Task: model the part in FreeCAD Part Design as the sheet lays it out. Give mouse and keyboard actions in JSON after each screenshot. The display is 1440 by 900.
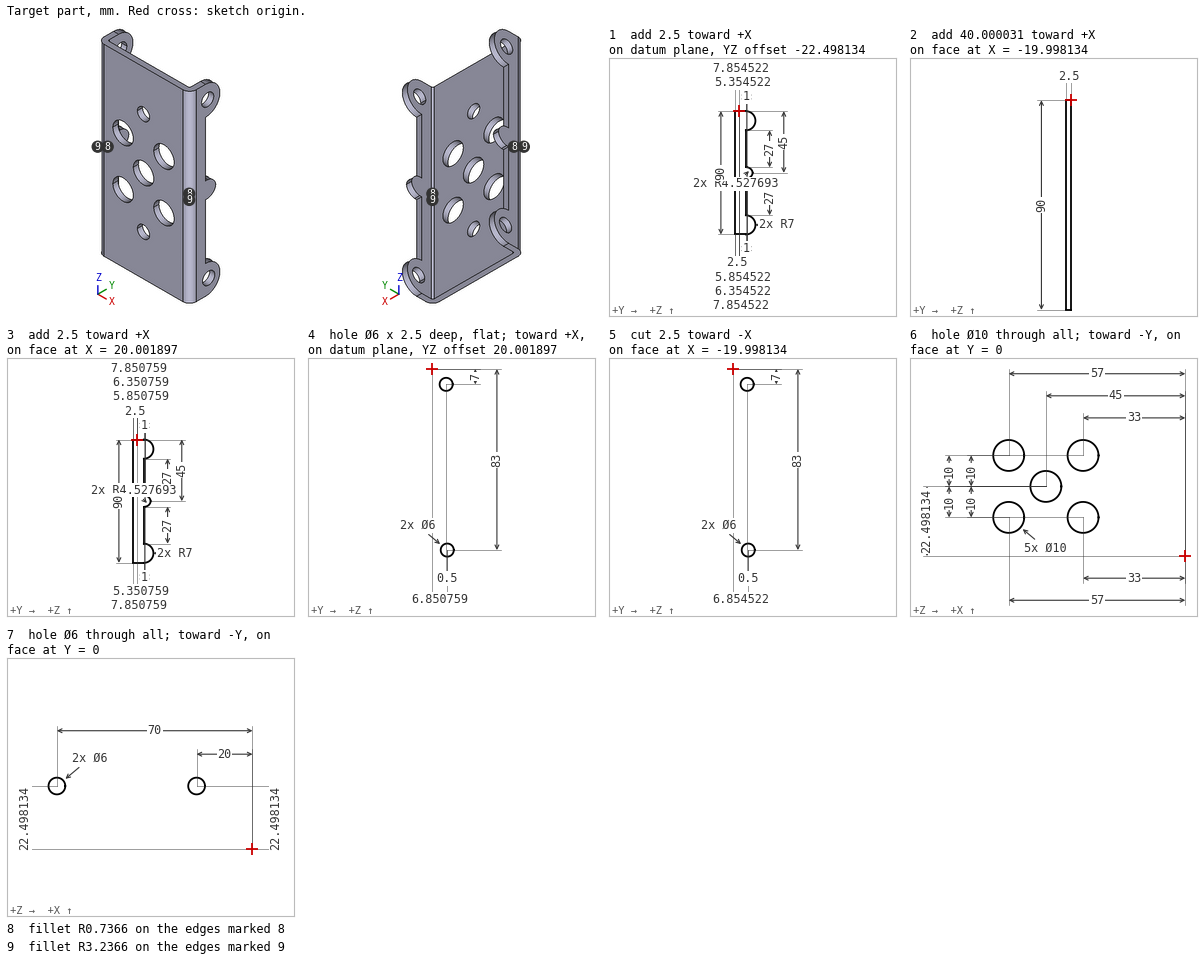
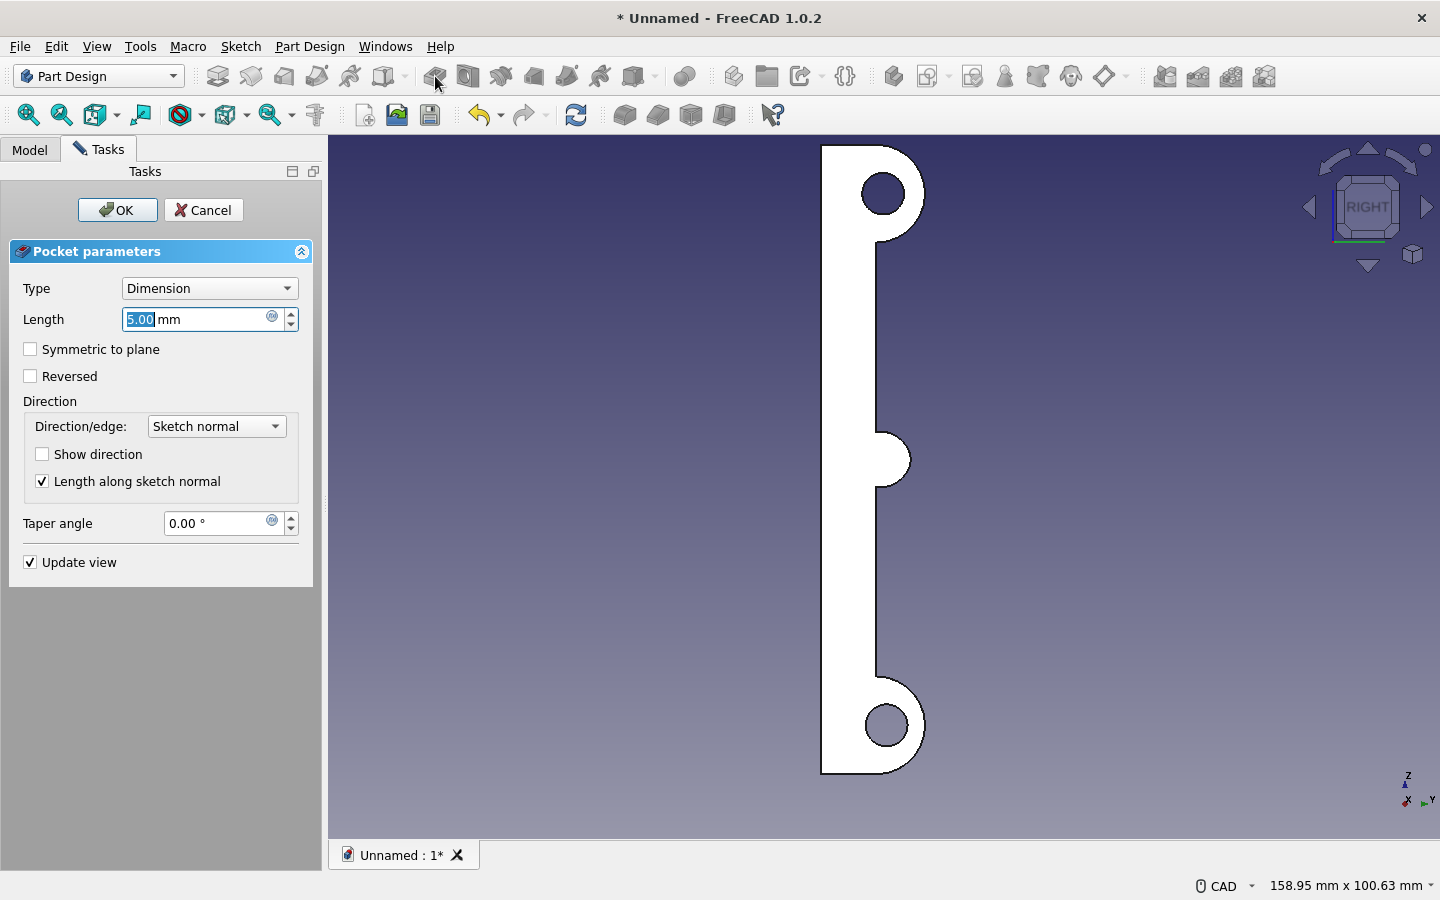
{"action": "type", "text": "2.5"}
{"action": "key", "text": "Tab"}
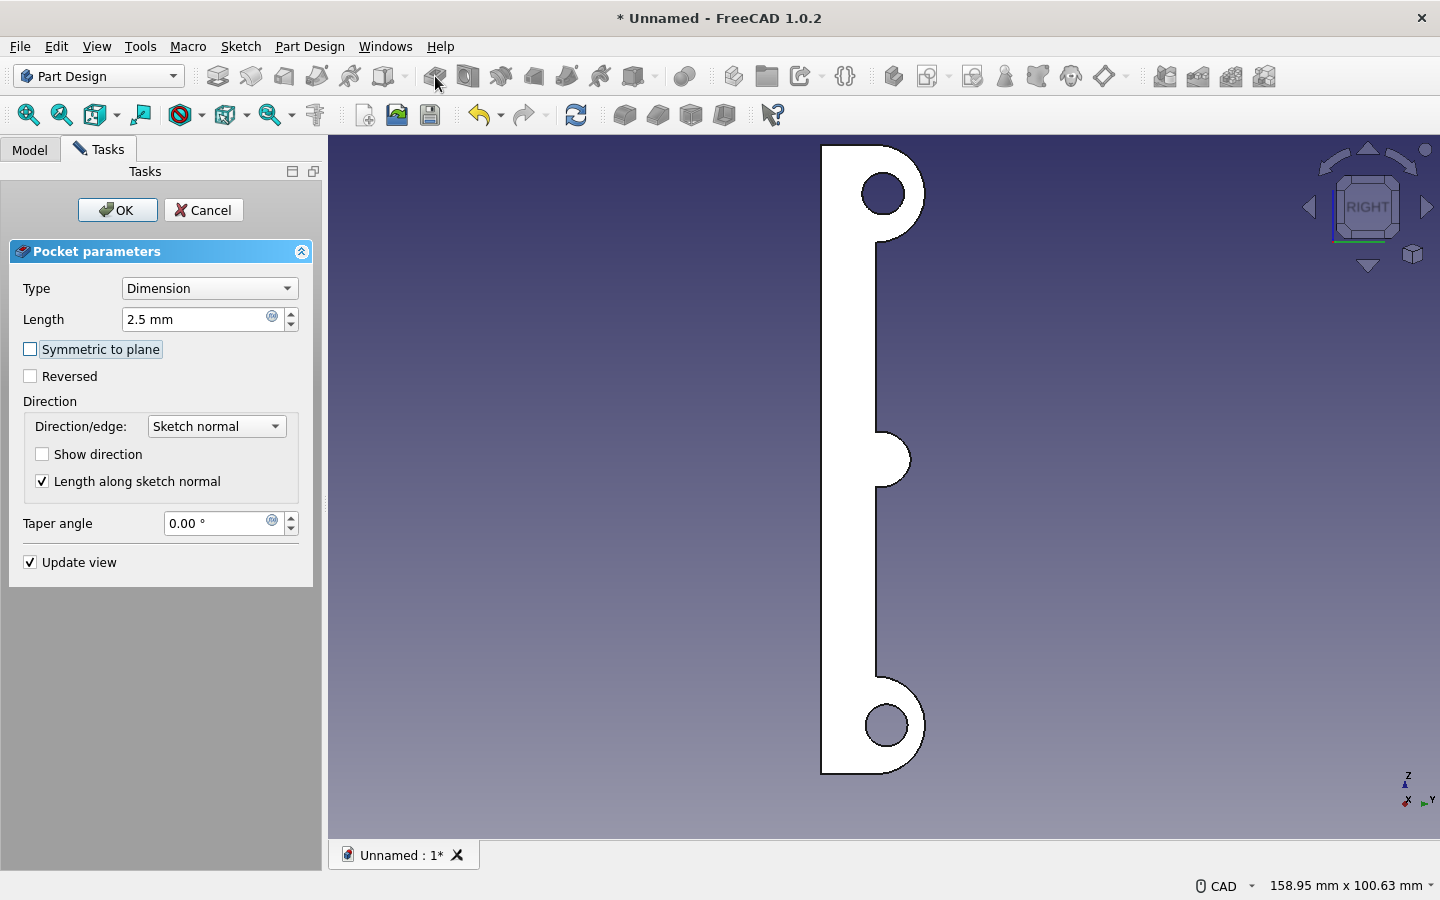
{"action": "left_click", "coordinate": [118, 210]}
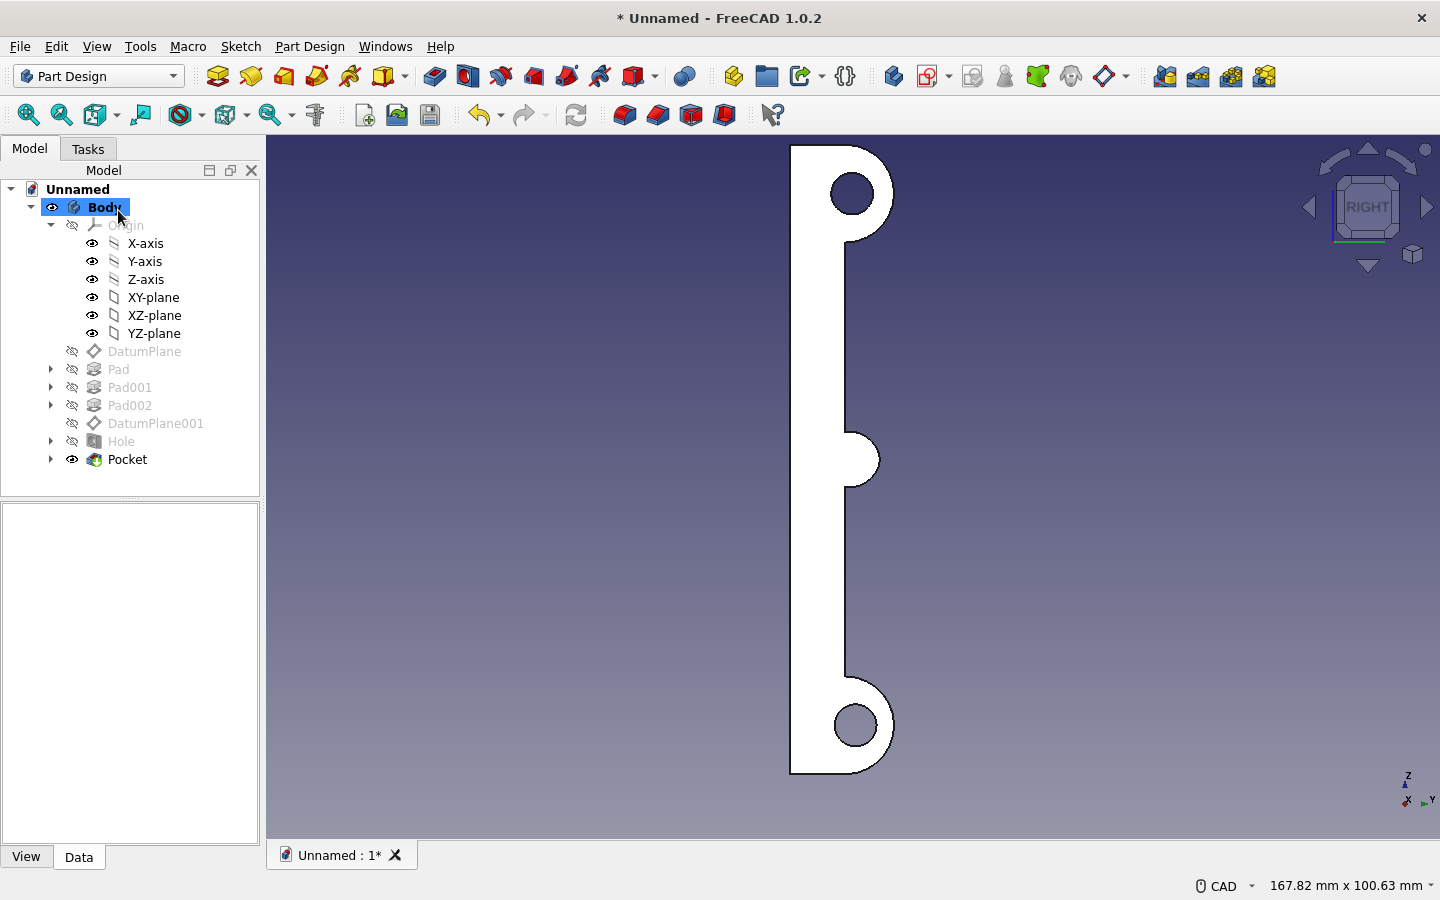
{"action": "key", "text": "4"}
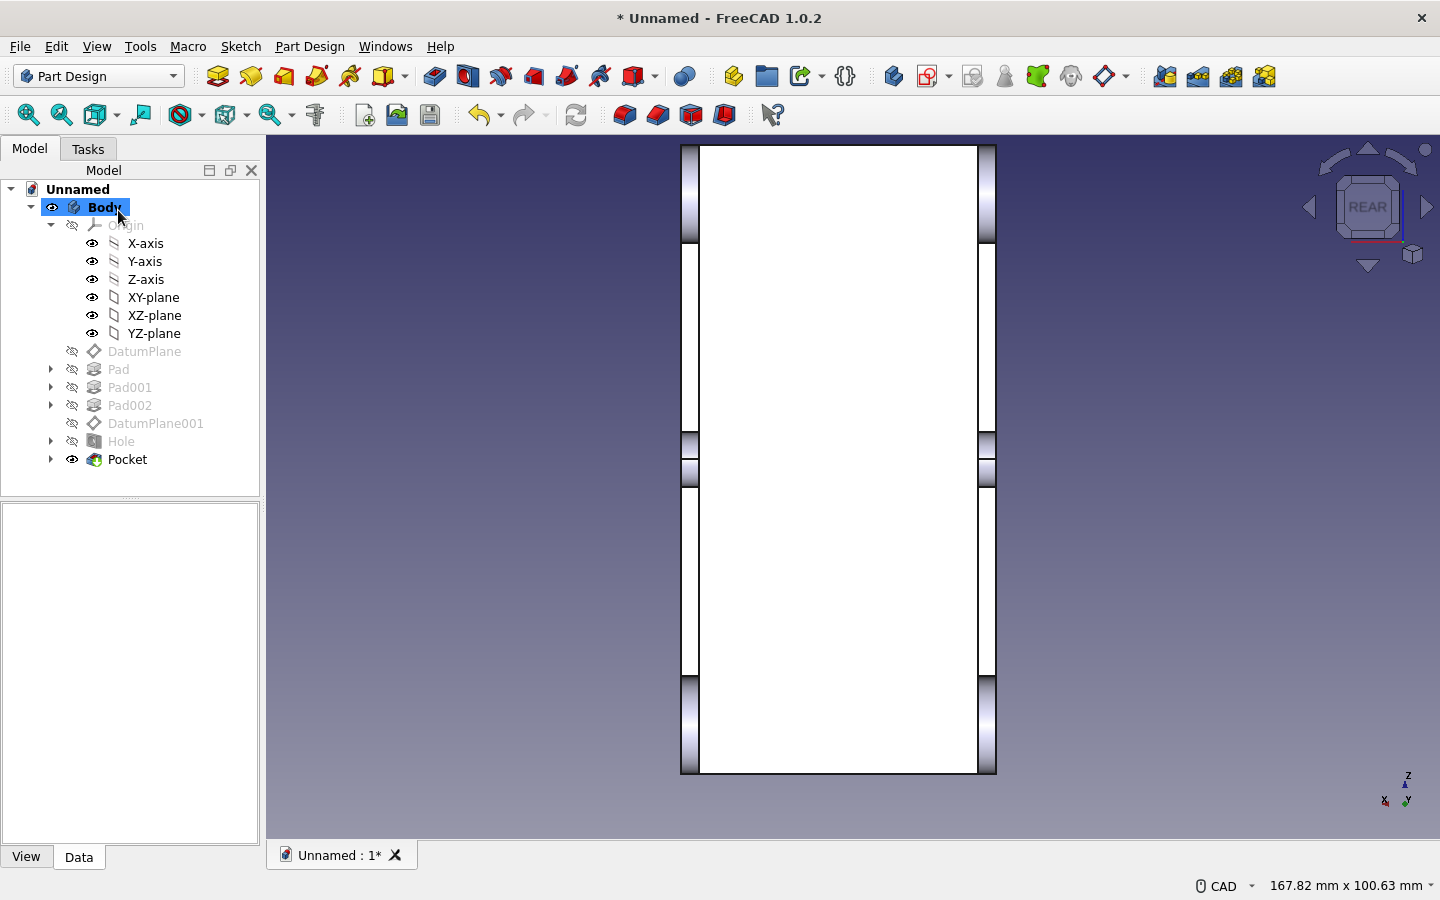
{"action": "left_click", "coordinate": [838, 369]}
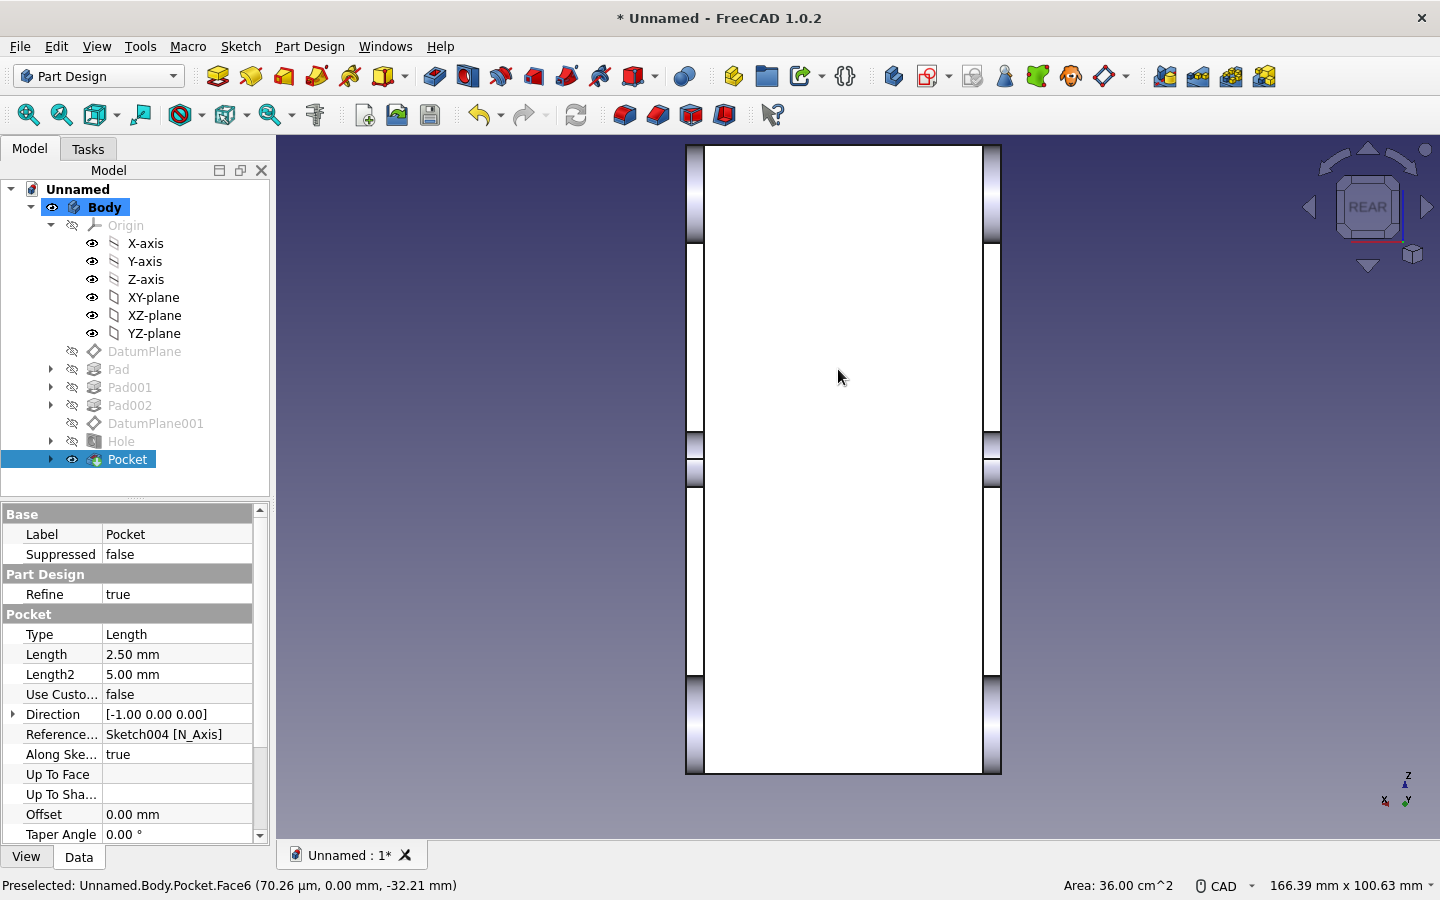
{"action": "left_click", "coordinate": [926, 76]}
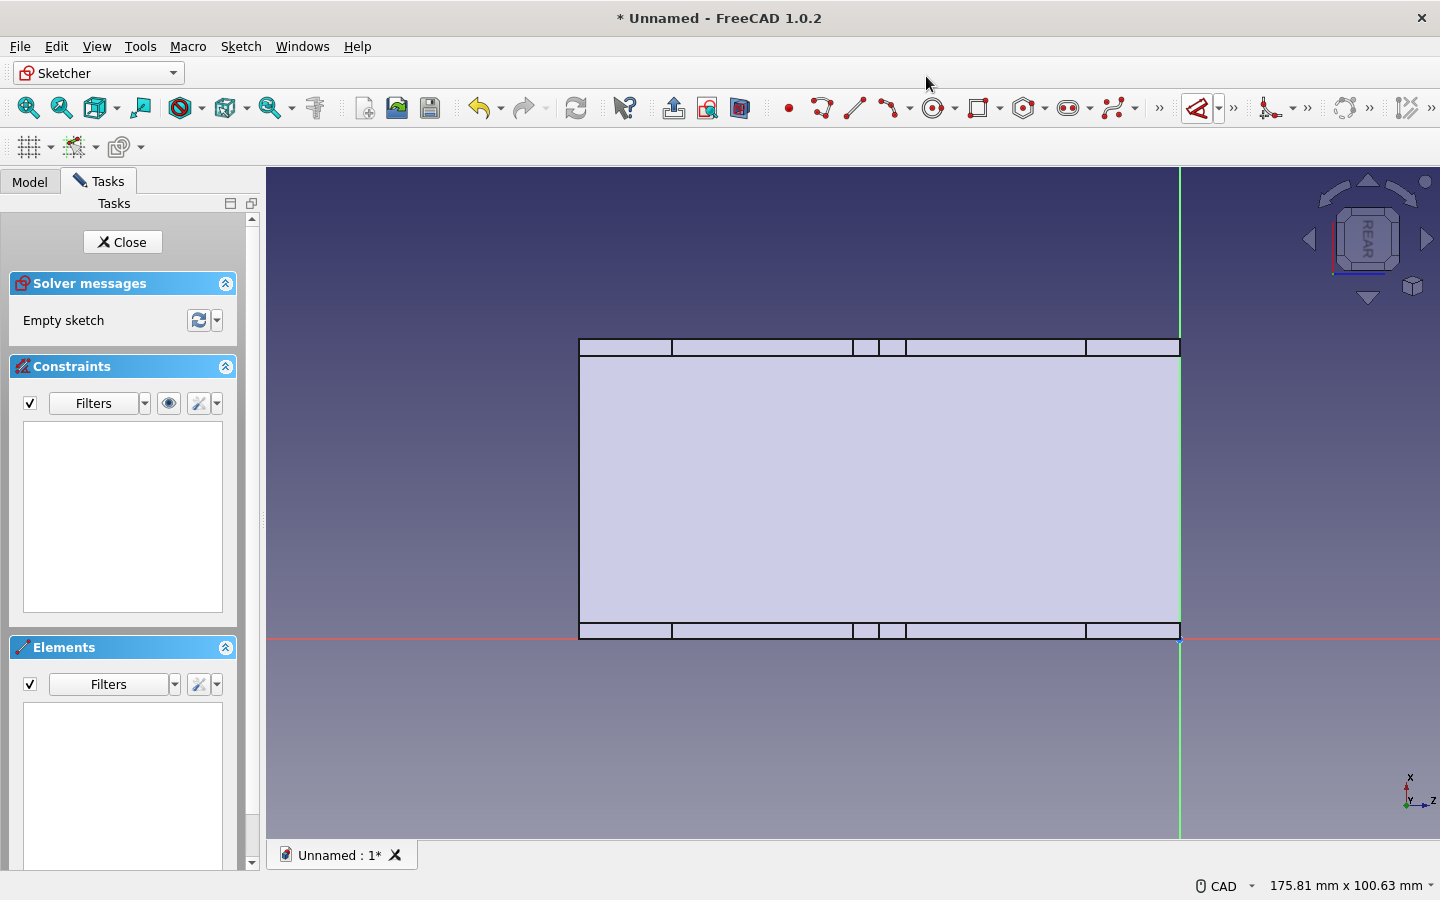
{"action": "left_click", "coordinate": [740, 108]}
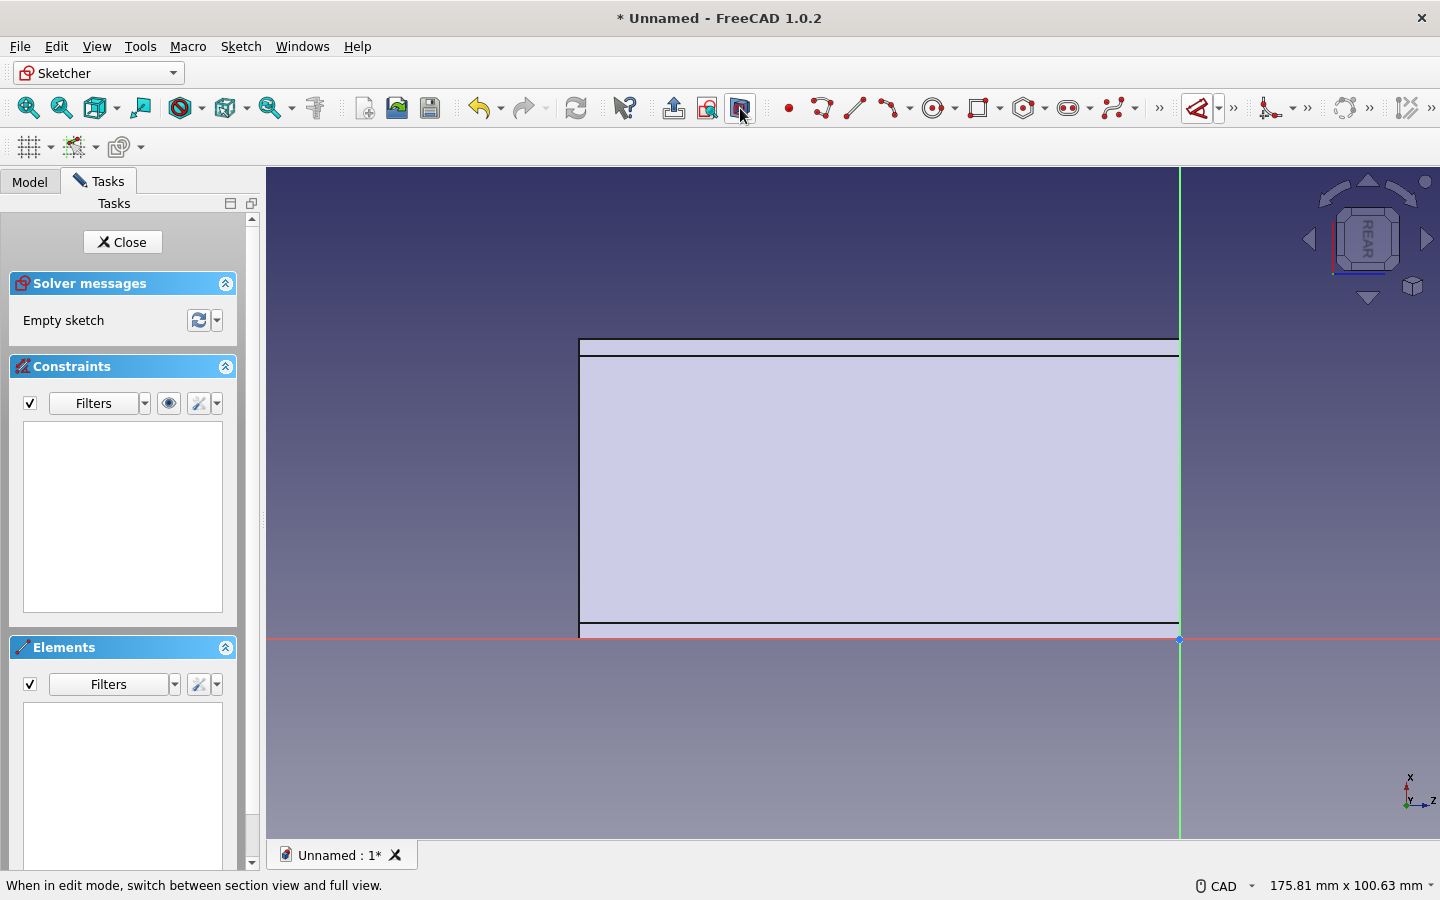
{"action": "scroll", "coordinate": [1202, 528], "scroll_direction": "up", "scroll_amount": 3}